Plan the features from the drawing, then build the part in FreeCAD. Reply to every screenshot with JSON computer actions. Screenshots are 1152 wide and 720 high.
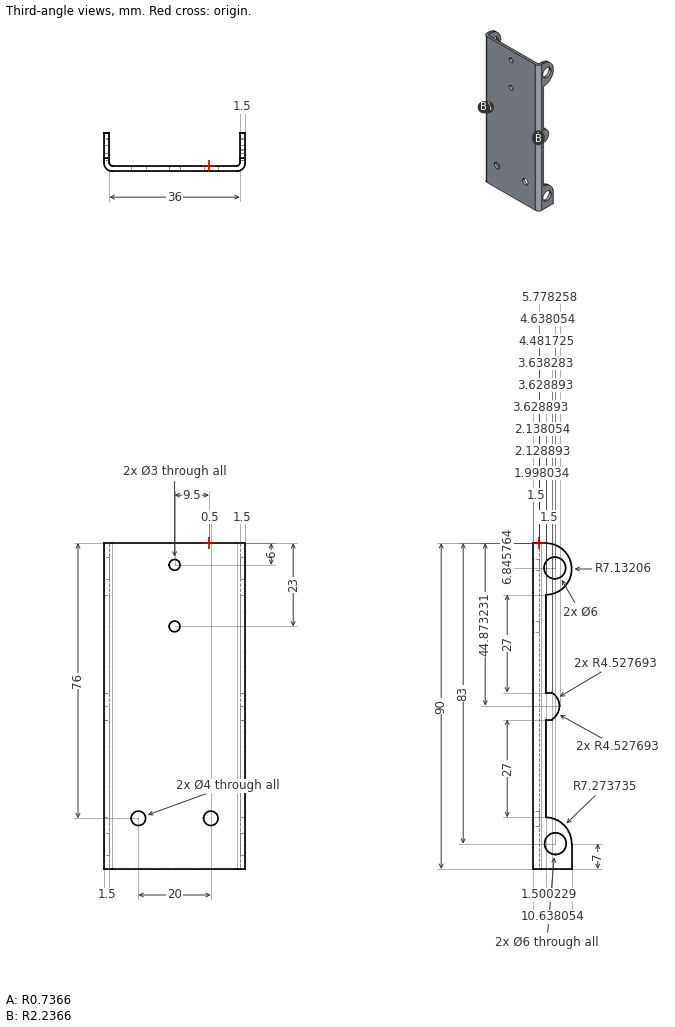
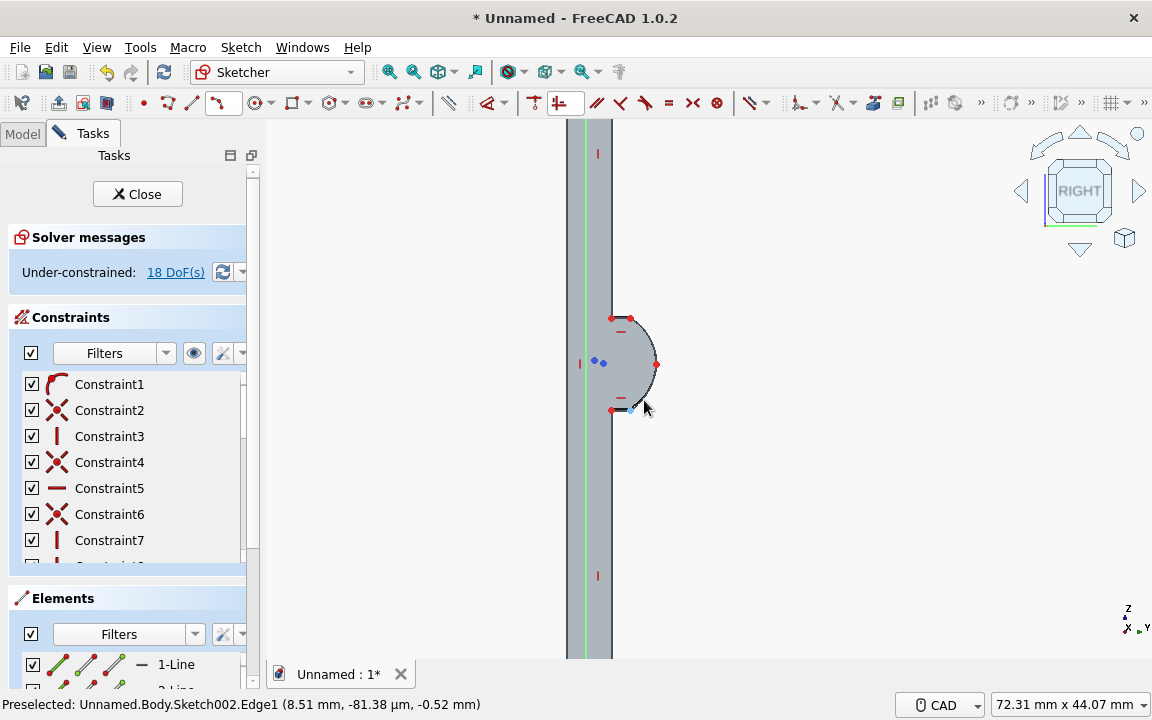
{"action": "left_click", "coordinate": [643, 399]}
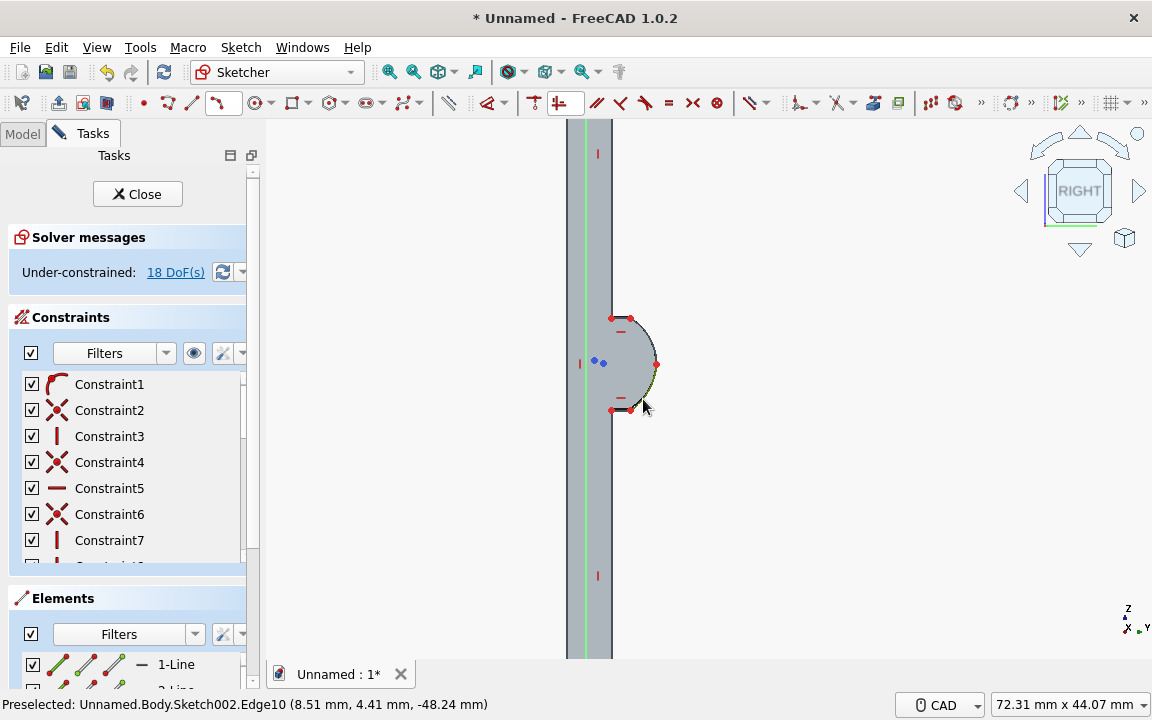
{"action": "left_click", "coordinate": [654, 348]}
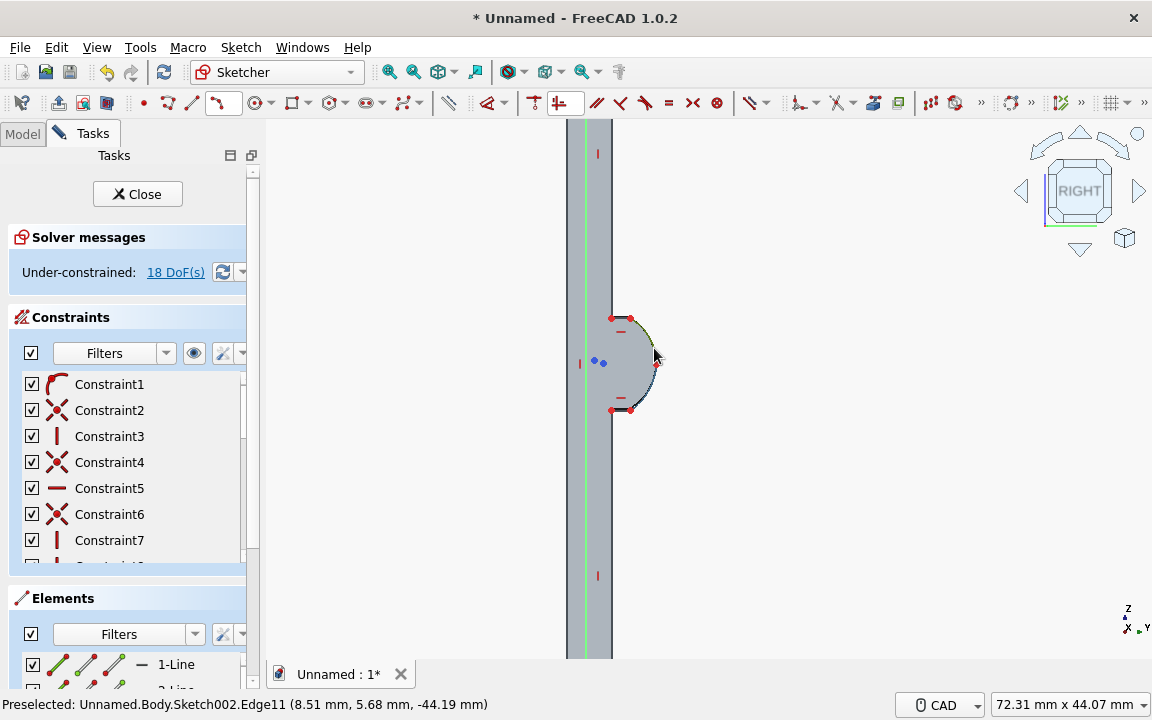
{"action": "key", "text": "e"}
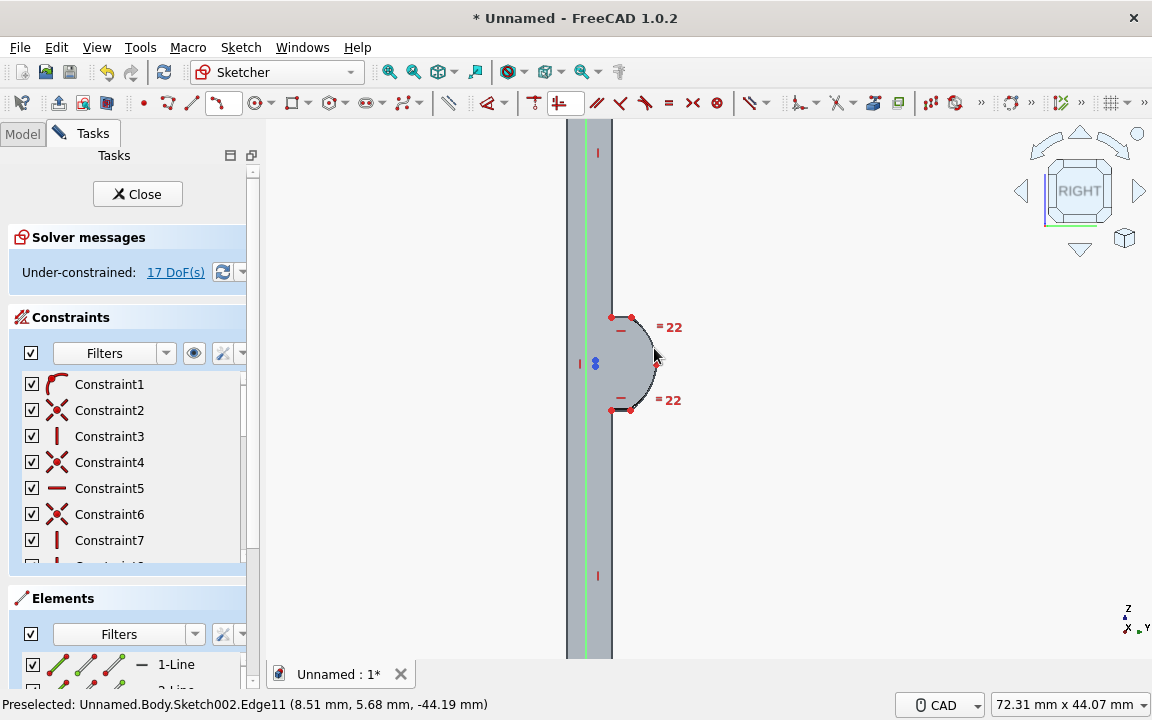
{"action": "key", "text": "d"}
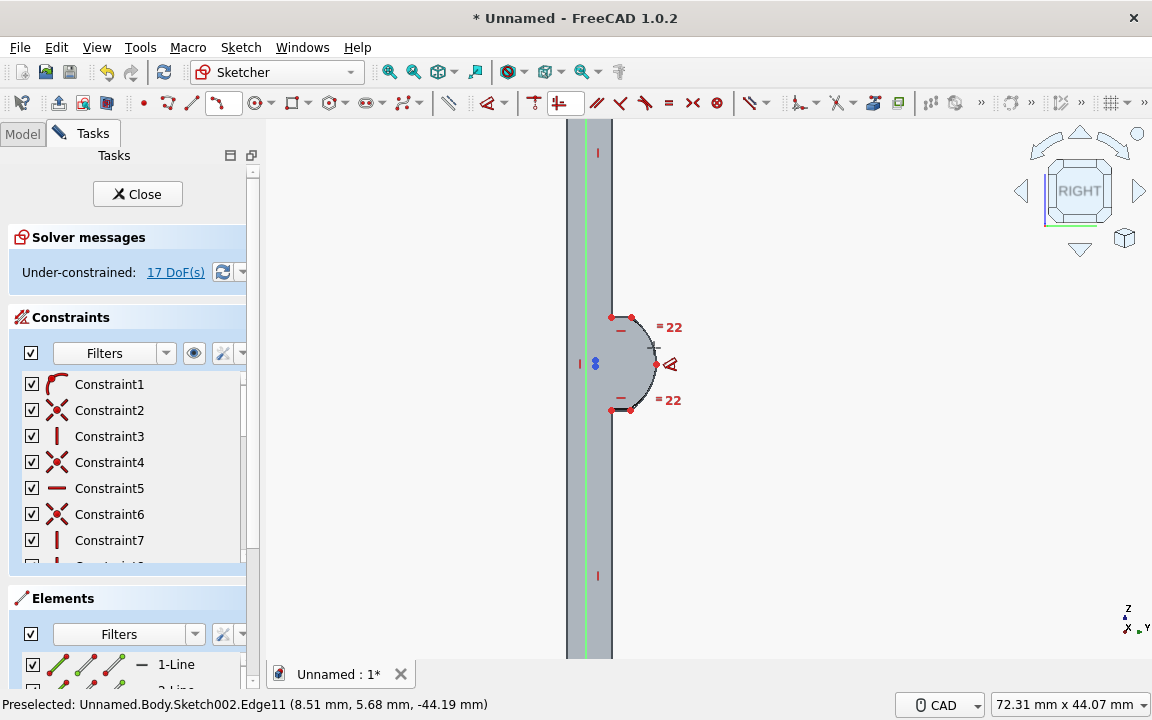
{"action": "scroll", "coordinate": [644, 400], "scroll_direction": "down", "scroll_amount": 6}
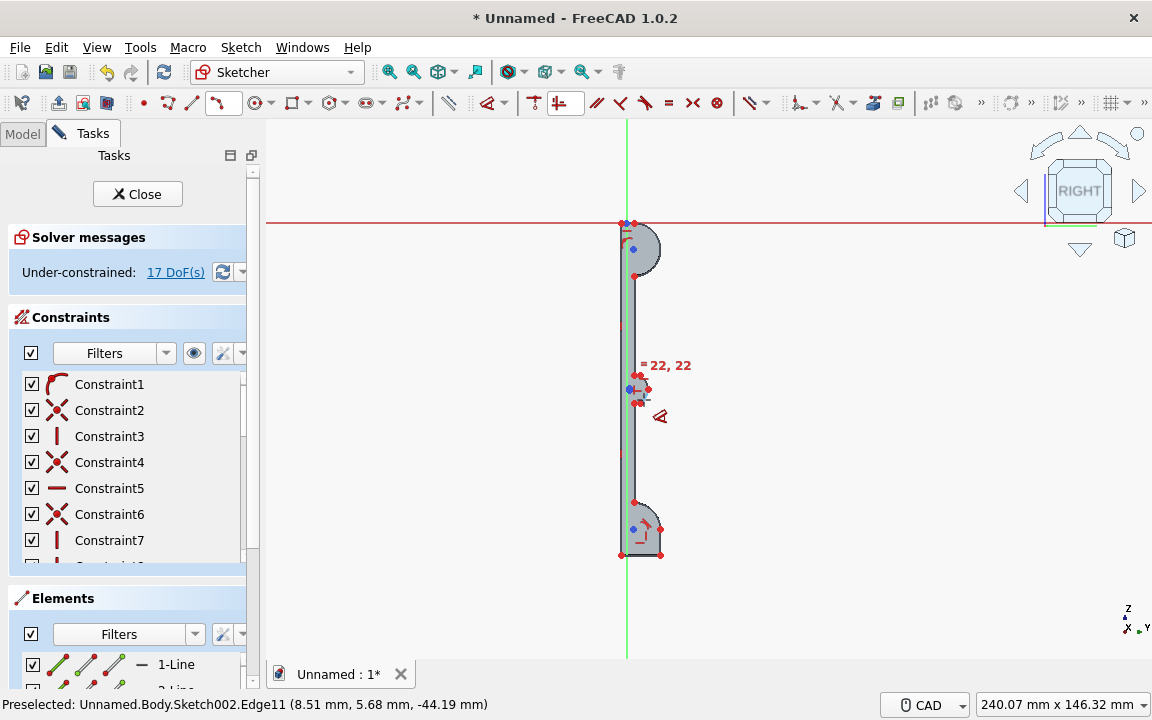
{"action": "scroll", "coordinate": [658, 518], "scroll_direction": "up", "scroll_amount": 2}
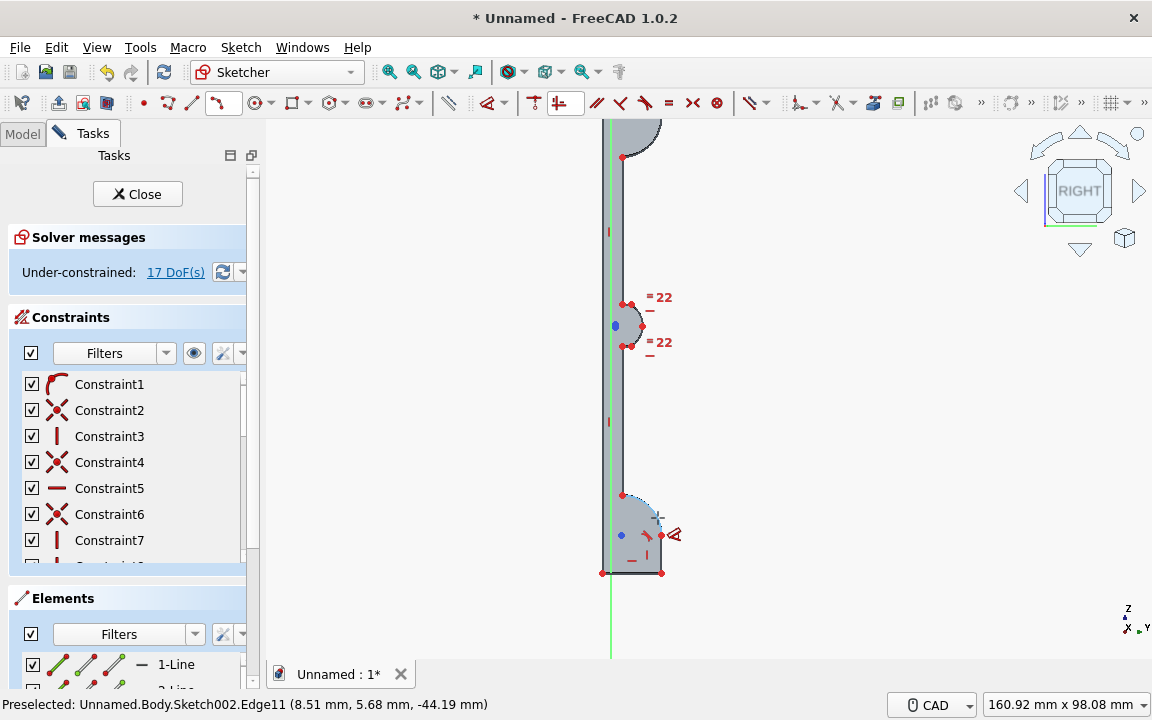
{"action": "left_click", "coordinate": [657, 518]}
{"action": "left_click", "coordinate": [686, 504]}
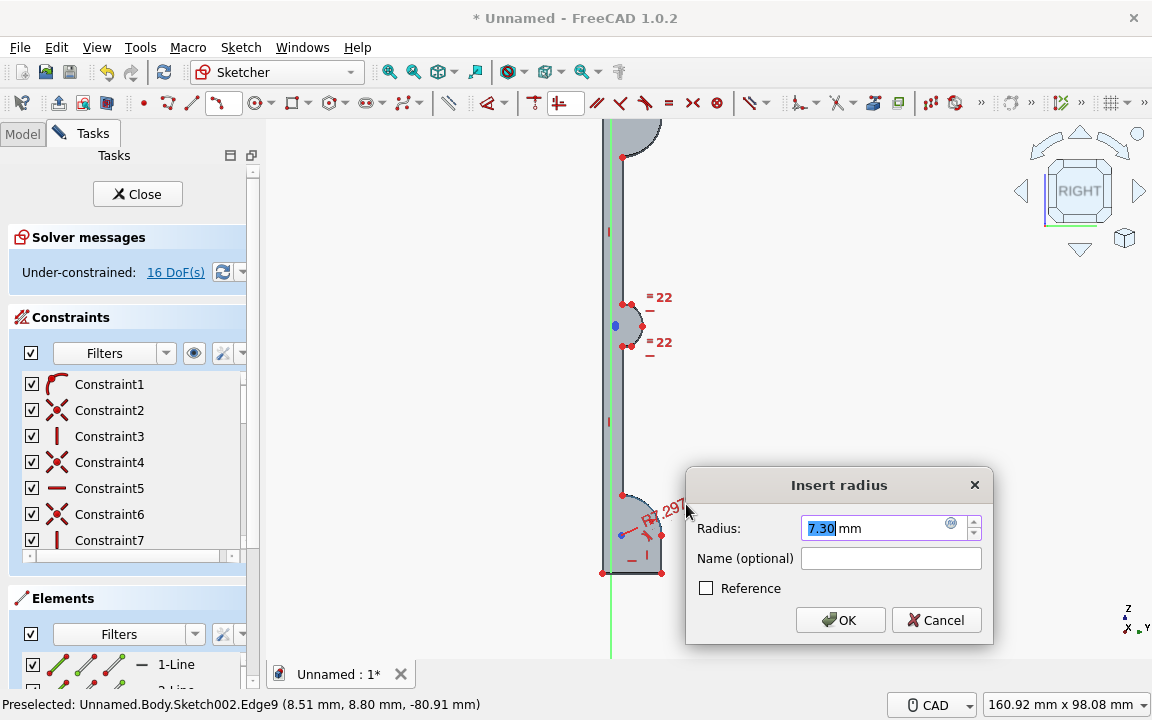
{"action": "type", "text": "7.273735"}
{"action": "key", "text": "Return"}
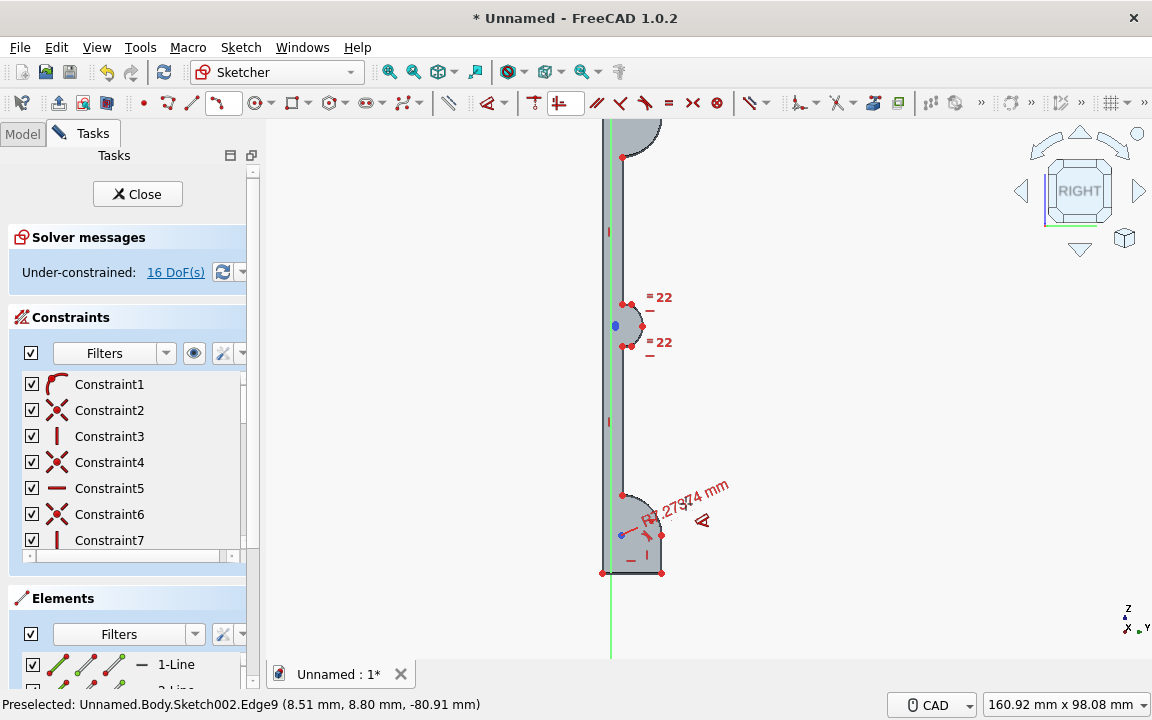
{"action": "scroll", "coordinate": [639, 338], "scroll_direction": "up", "scroll_amount": 3}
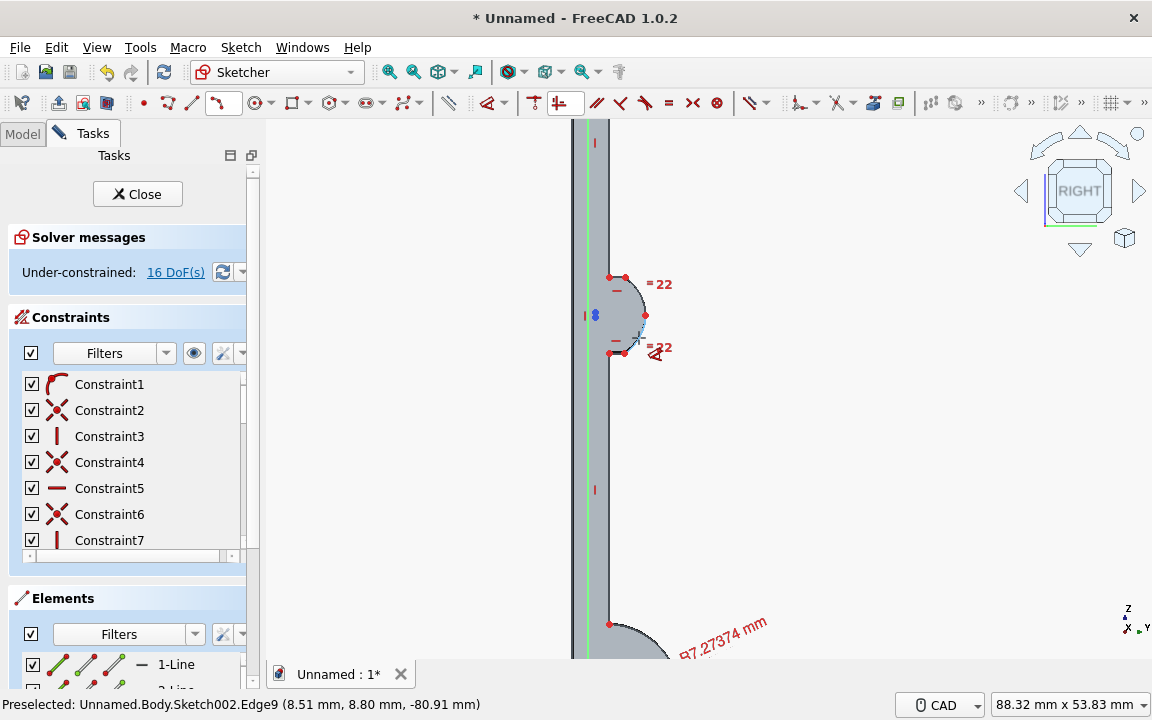
{"action": "left_click", "coordinate": [640, 337]}
{"action": "left_click", "coordinate": [668, 352]}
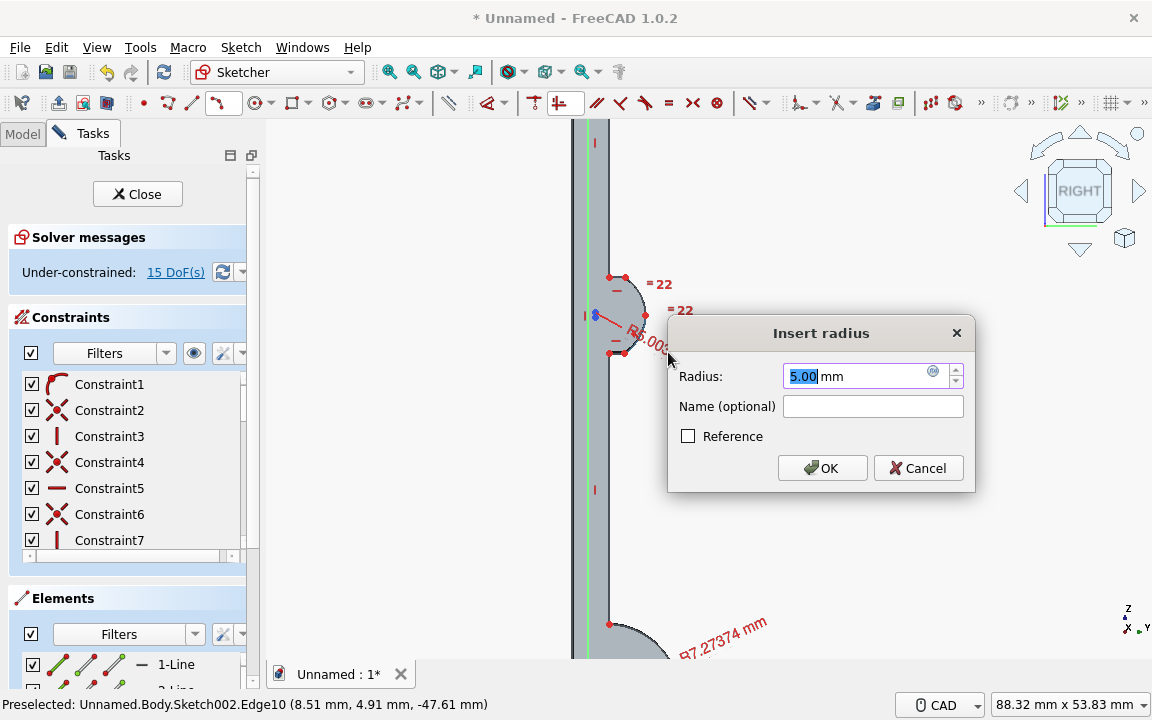
{"action": "type", "text": "4.527693"}
{"action": "key", "text": "Return"}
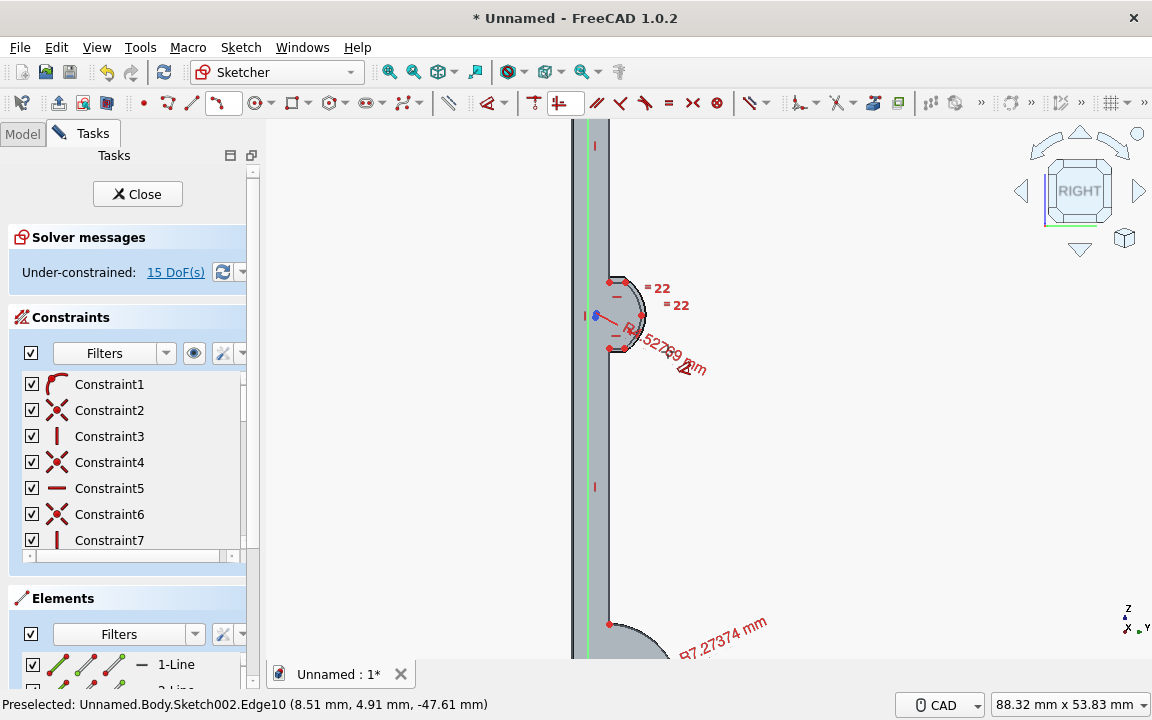
{"action": "scroll", "coordinate": [649, 432], "scroll_direction": "down", "scroll_amount": 5}